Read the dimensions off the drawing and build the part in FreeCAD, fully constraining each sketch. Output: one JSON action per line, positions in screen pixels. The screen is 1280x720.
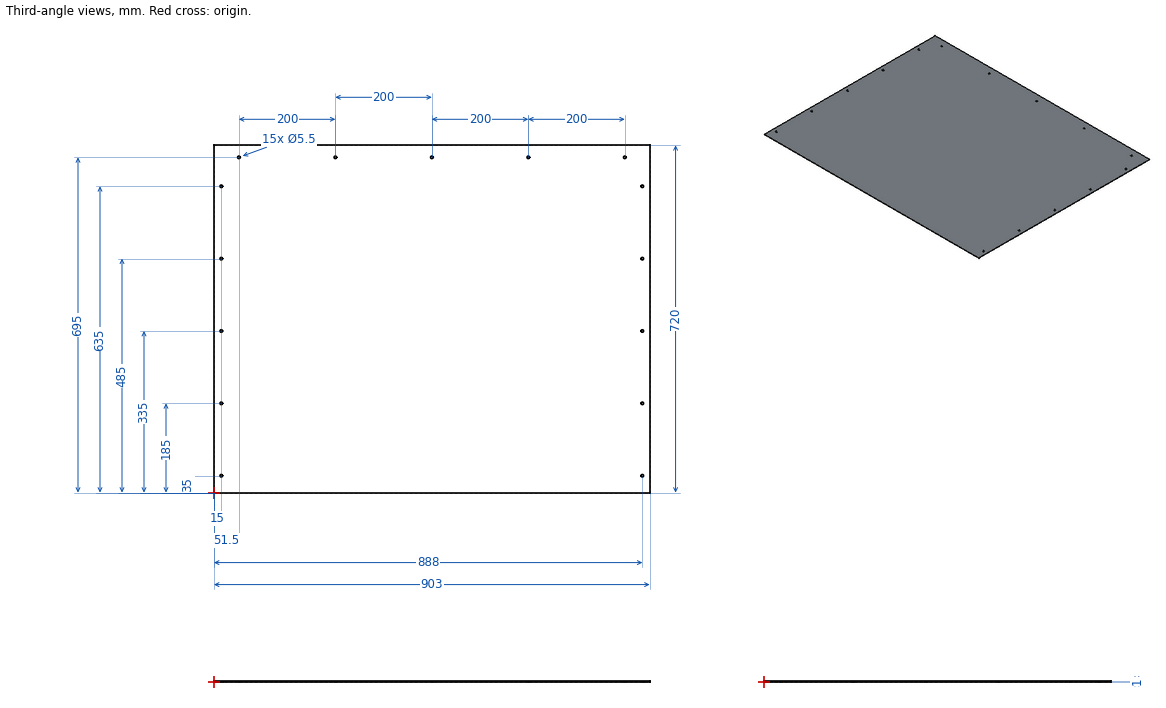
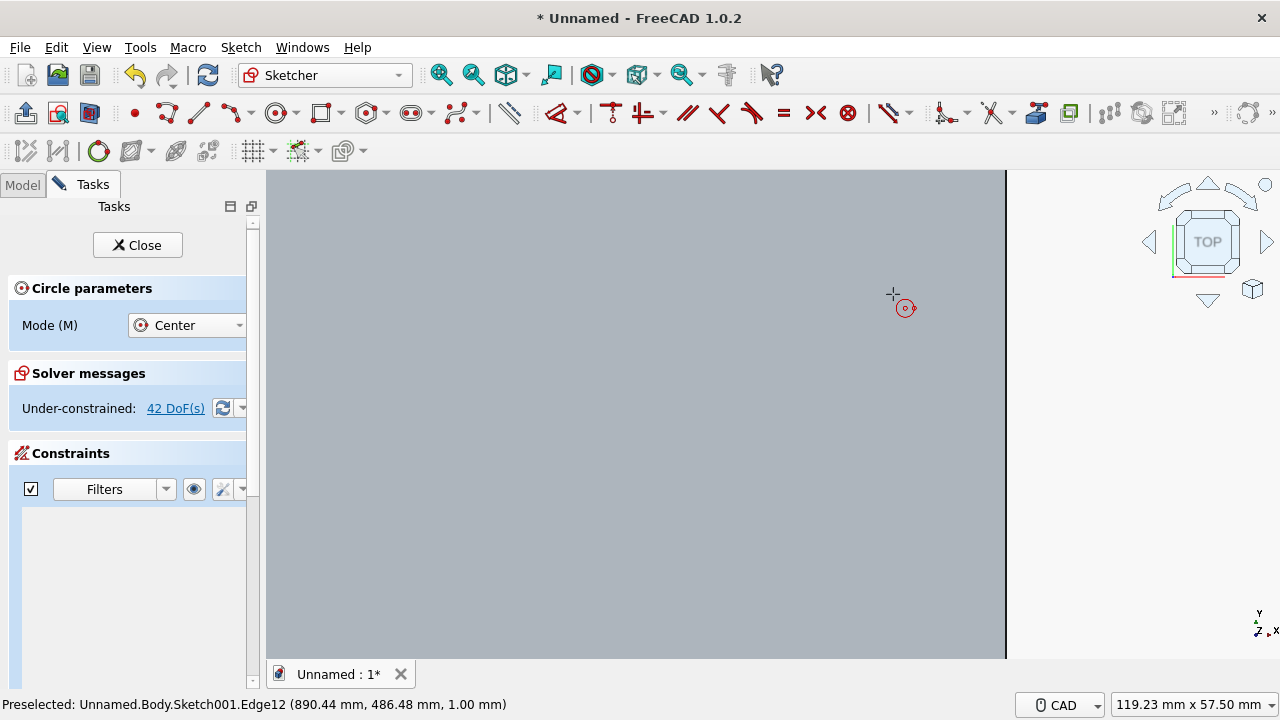
{"action": "scroll", "coordinate": [893, 293], "scroll_direction": "down", "scroll_amount": 15}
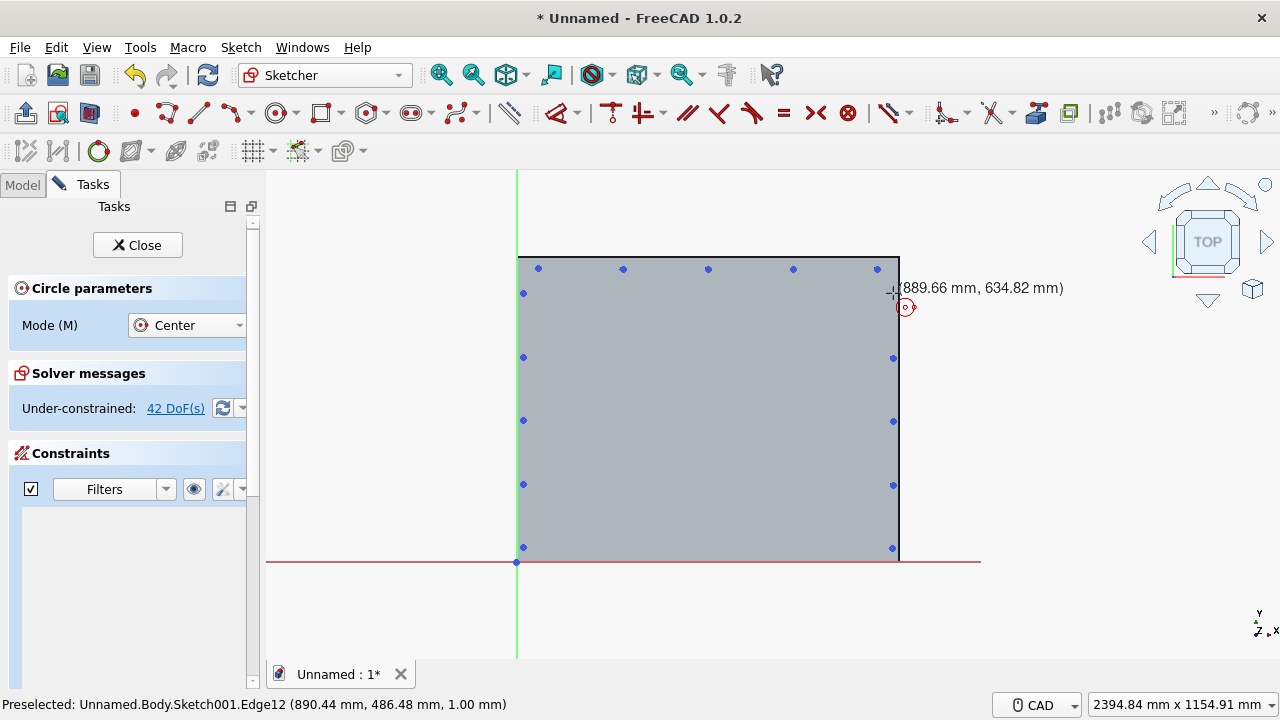
{"action": "left_click", "coordinate": [893, 293]}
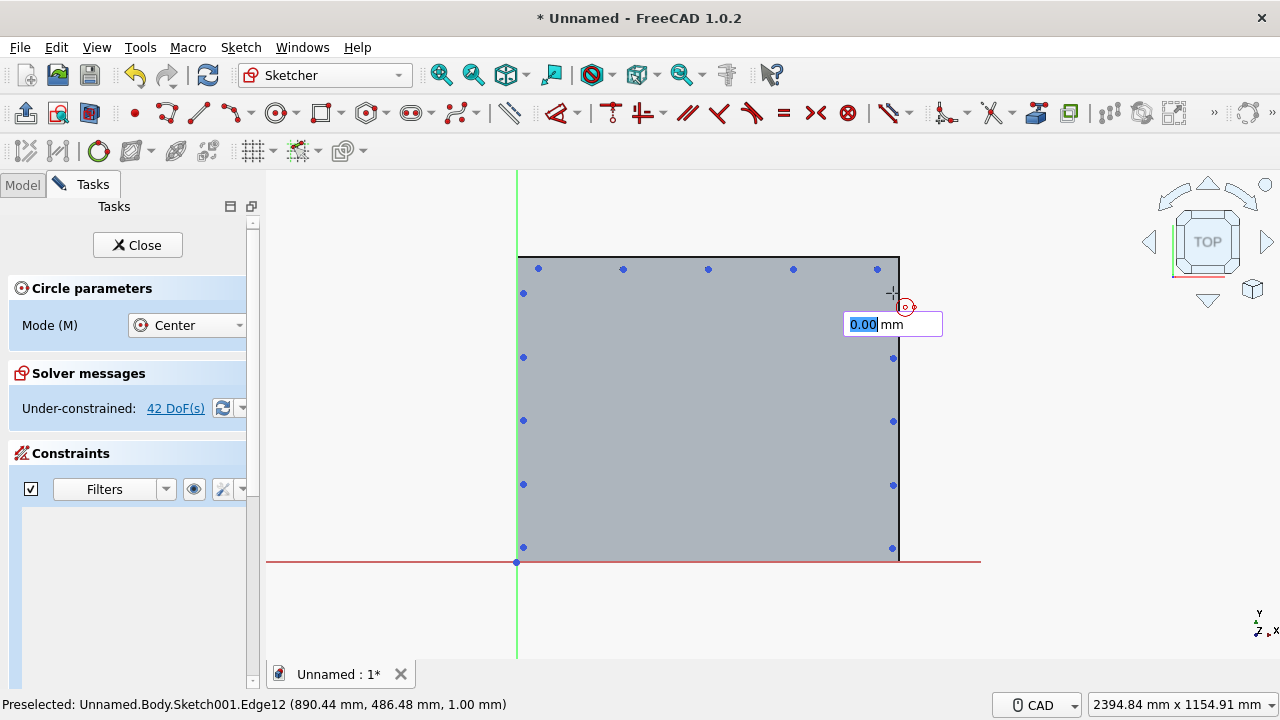
{"action": "scroll", "coordinate": [894, 292], "scroll_direction": "up", "scroll_amount": 14}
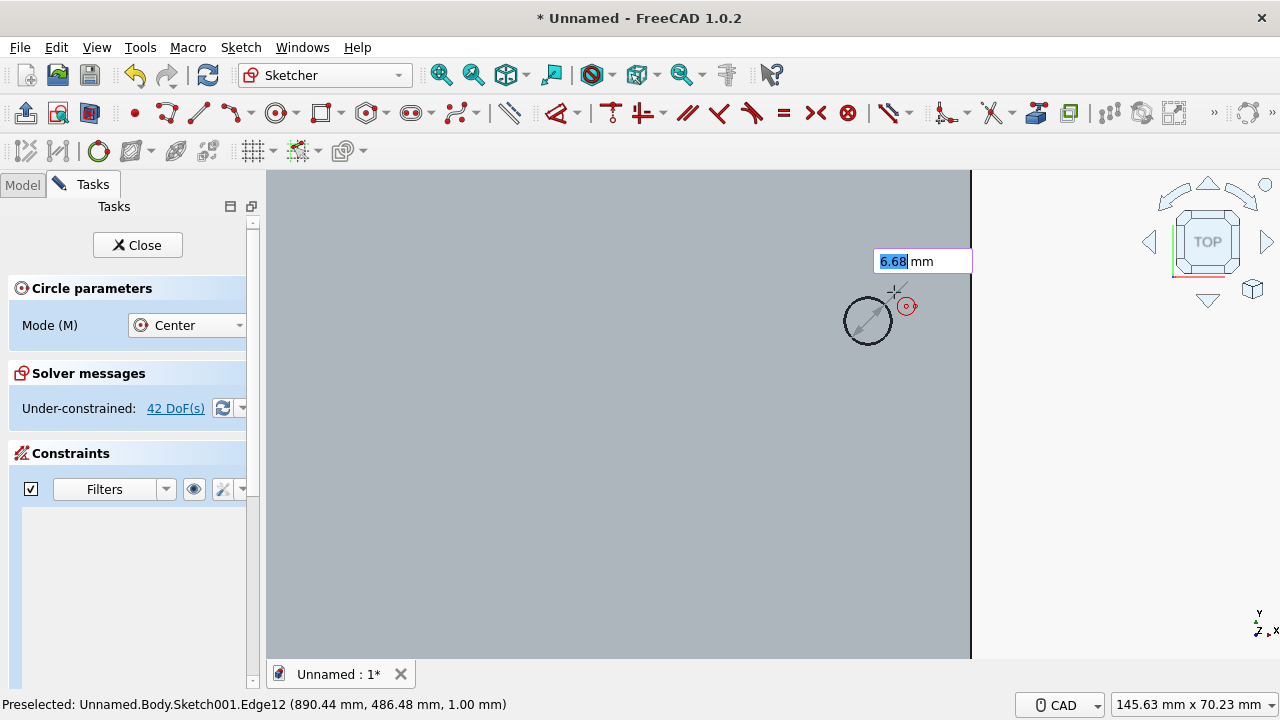
{"action": "left_click", "coordinate": [880, 295]}
{"action": "key", "text": "Escape"}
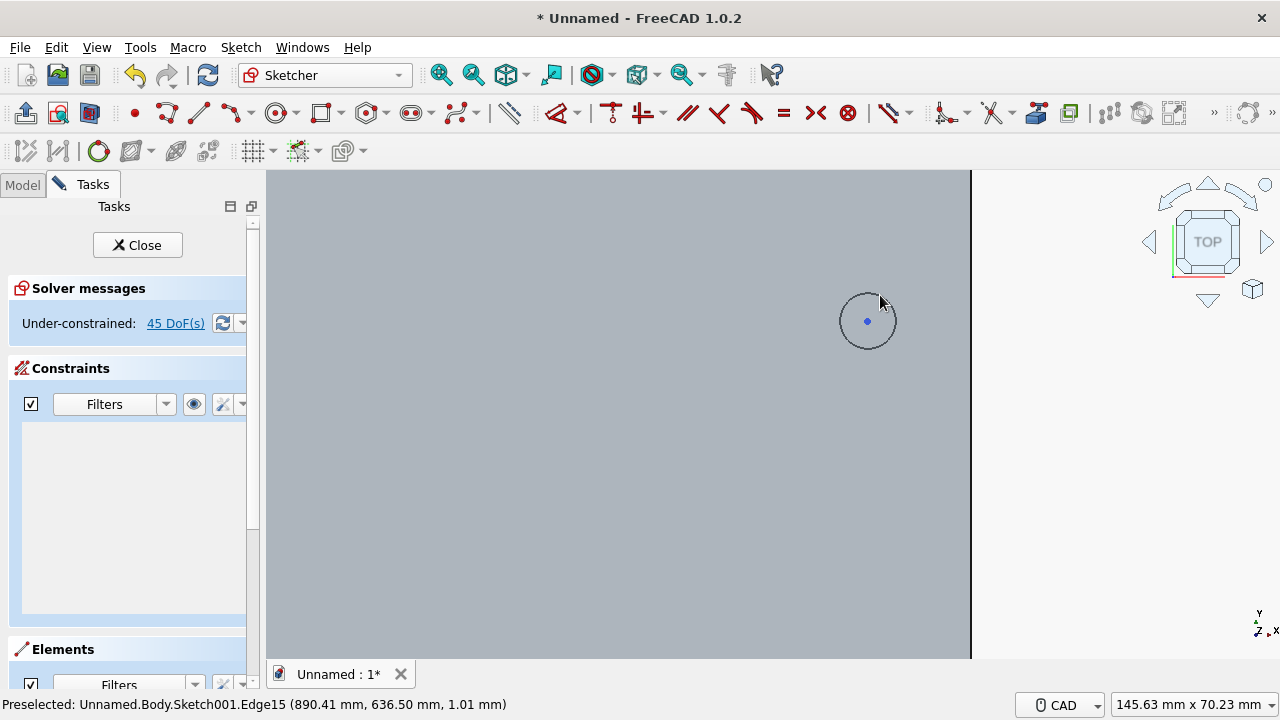
{"action": "scroll", "coordinate": [894, 292], "scroll_direction": "down", "scroll_amount": 14}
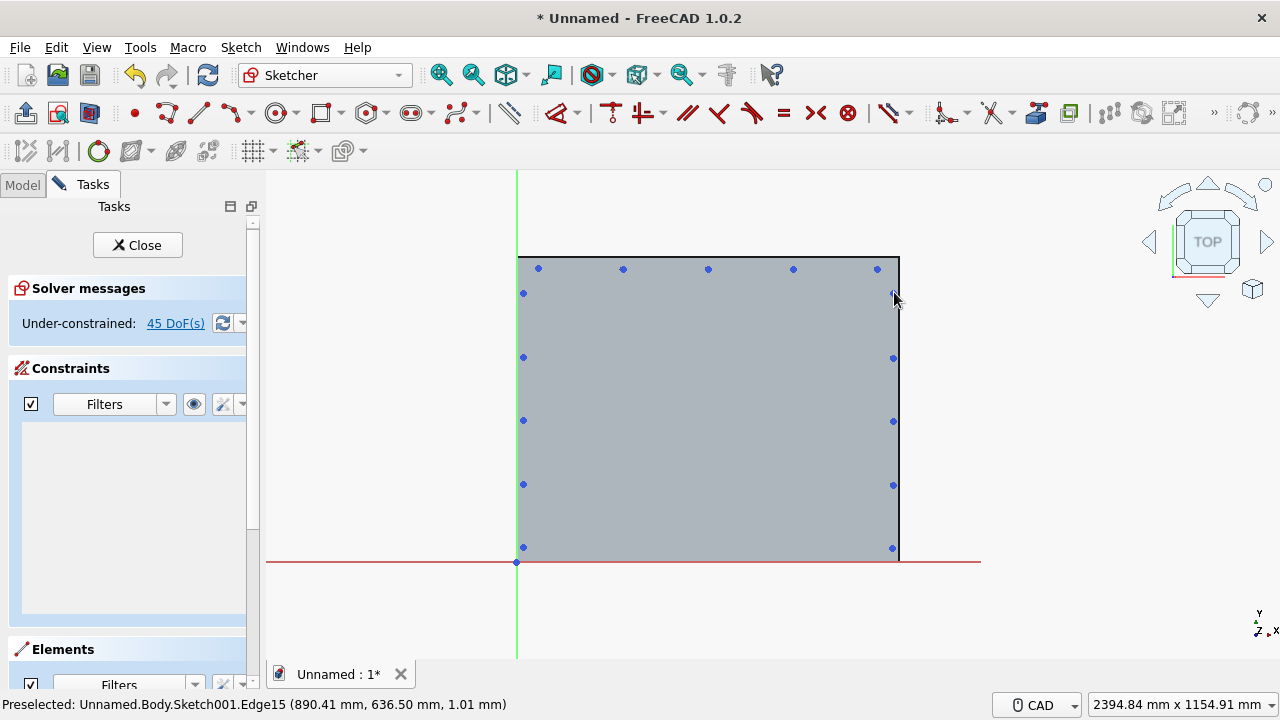
{"action": "scroll", "coordinate": [540, 267], "scroll_direction": "up", "scroll_amount": 10}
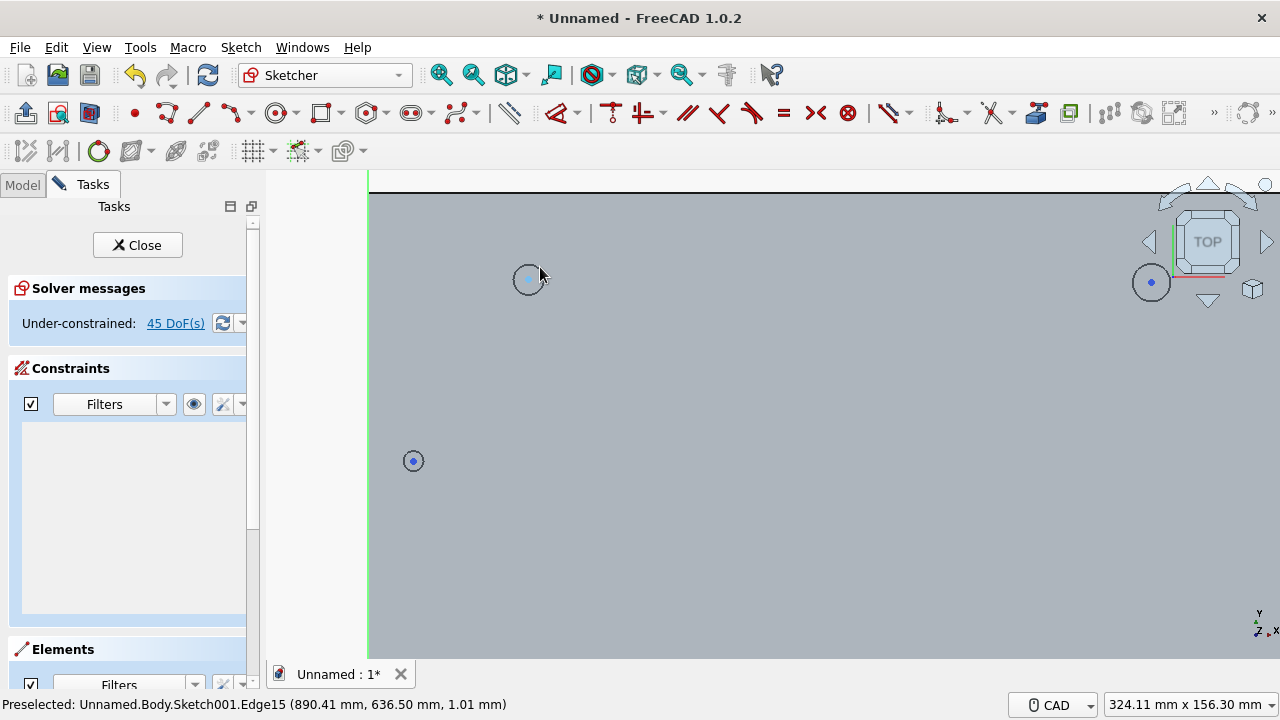
{"action": "left_click", "coordinate": [539, 269]}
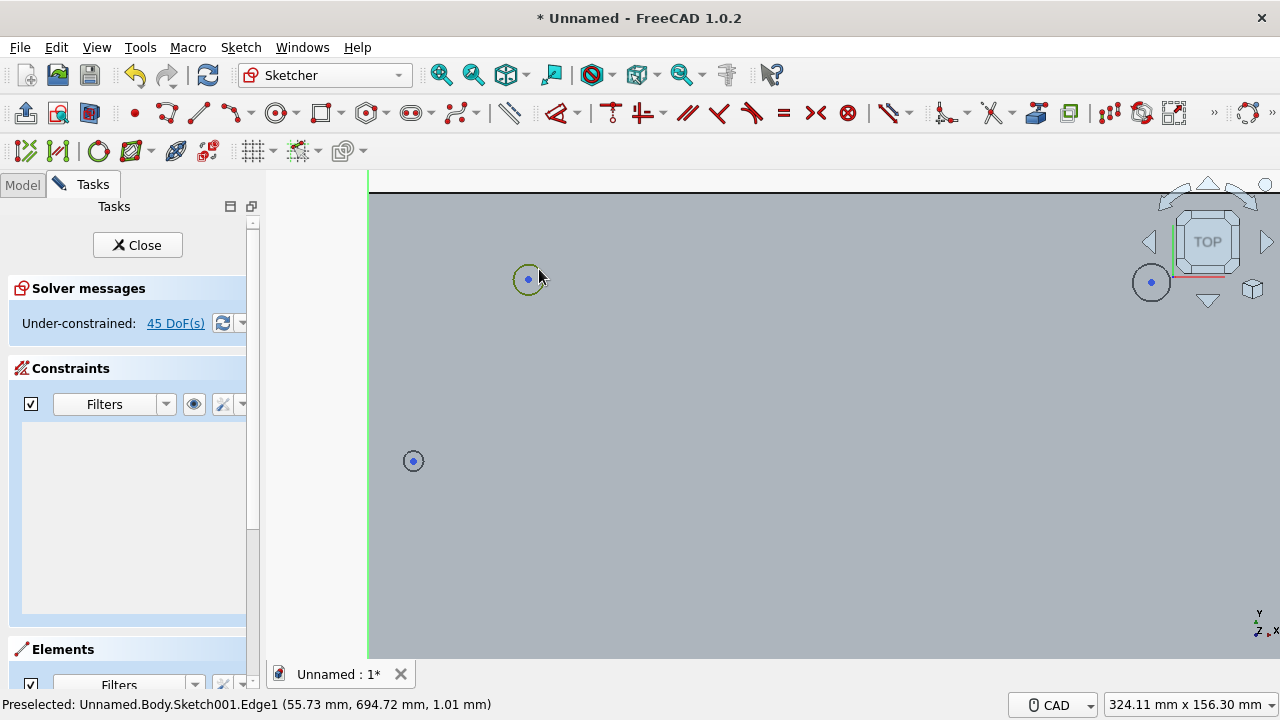
{"action": "scroll", "coordinate": [421, 454], "scroll_direction": "up", "scroll_amount": 2}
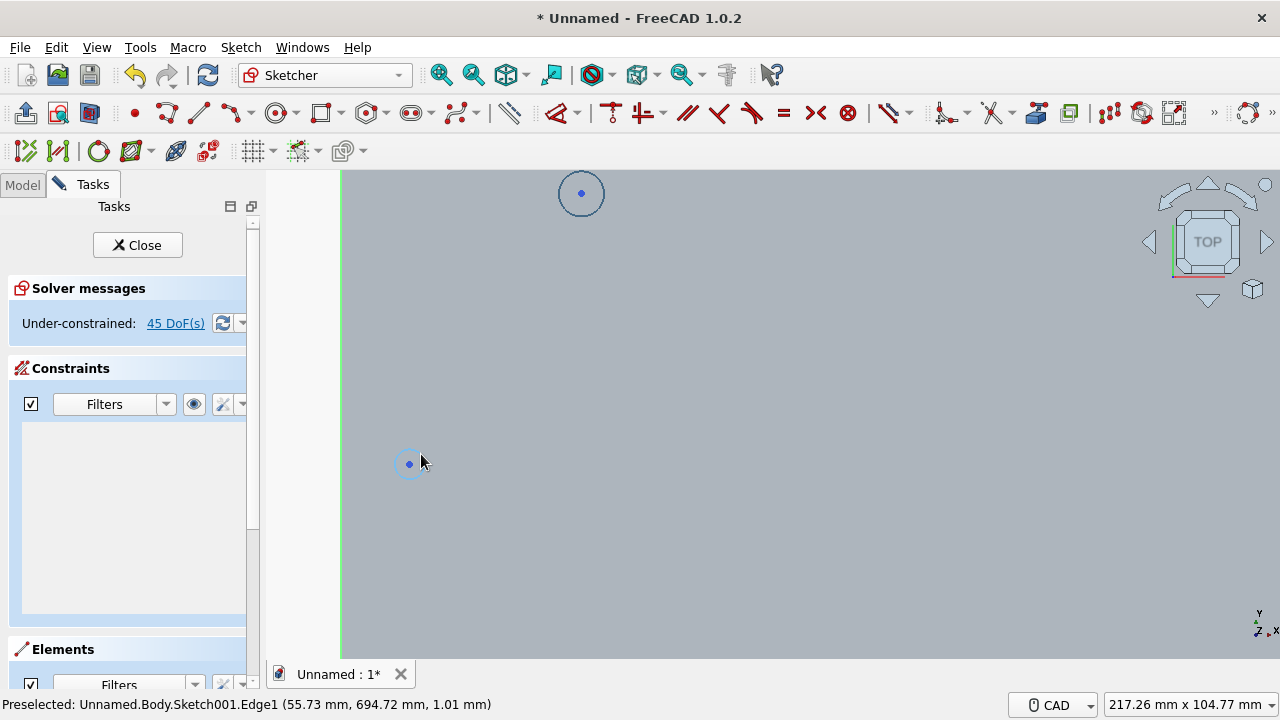
{"action": "left_click", "coordinate": [420, 454]}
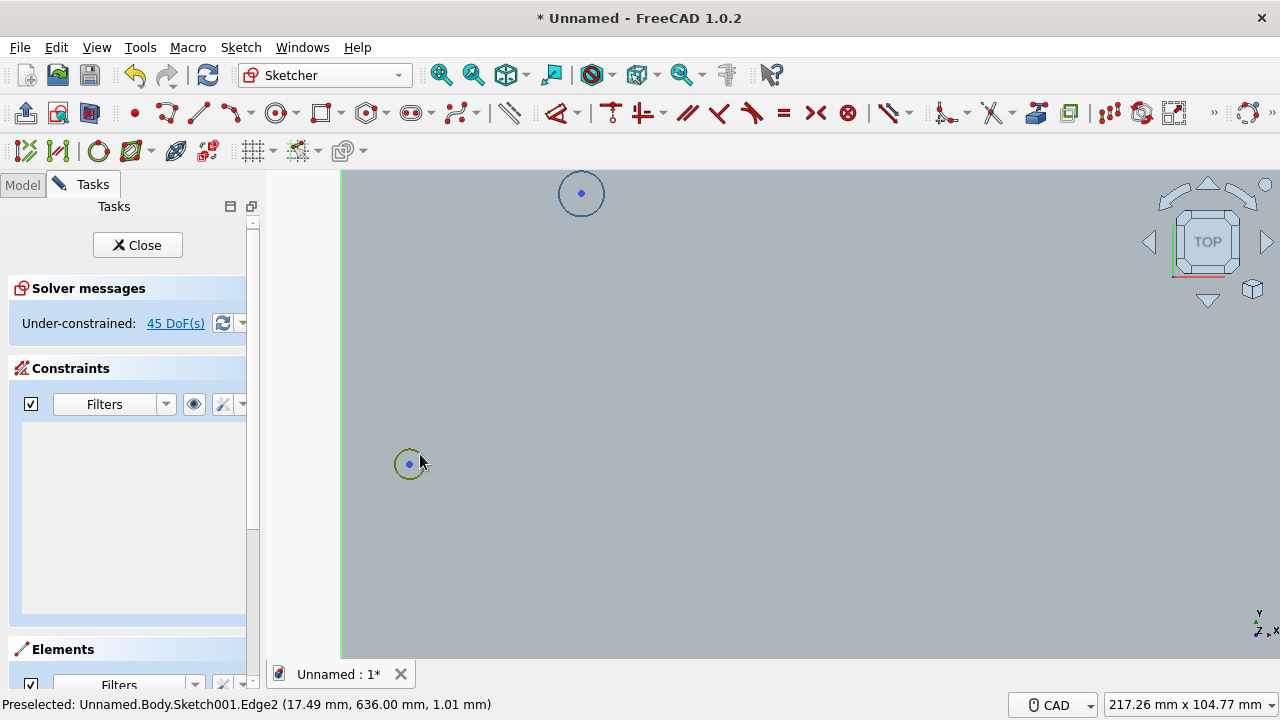
{"action": "scroll", "coordinate": [533, 277], "scroll_direction": "down", "scroll_amount": 12}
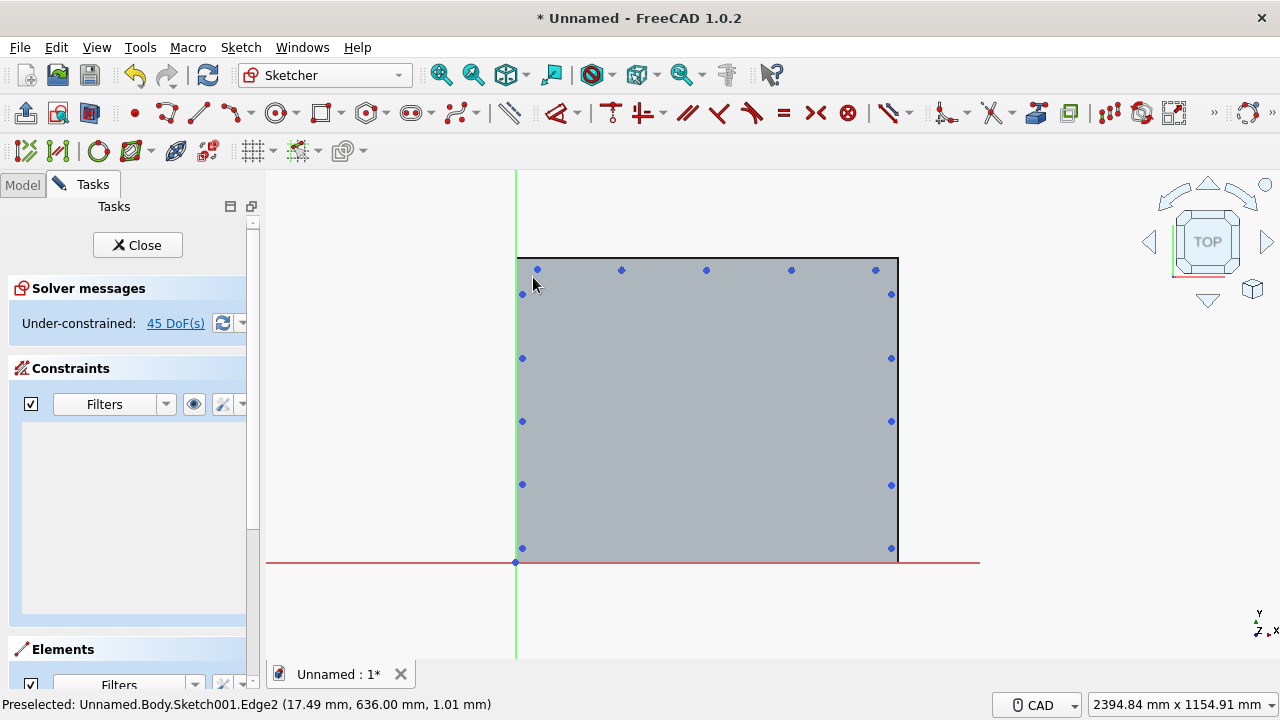
{"action": "scroll", "coordinate": [624, 268], "scroll_direction": "up", "scroll_amount": 9}